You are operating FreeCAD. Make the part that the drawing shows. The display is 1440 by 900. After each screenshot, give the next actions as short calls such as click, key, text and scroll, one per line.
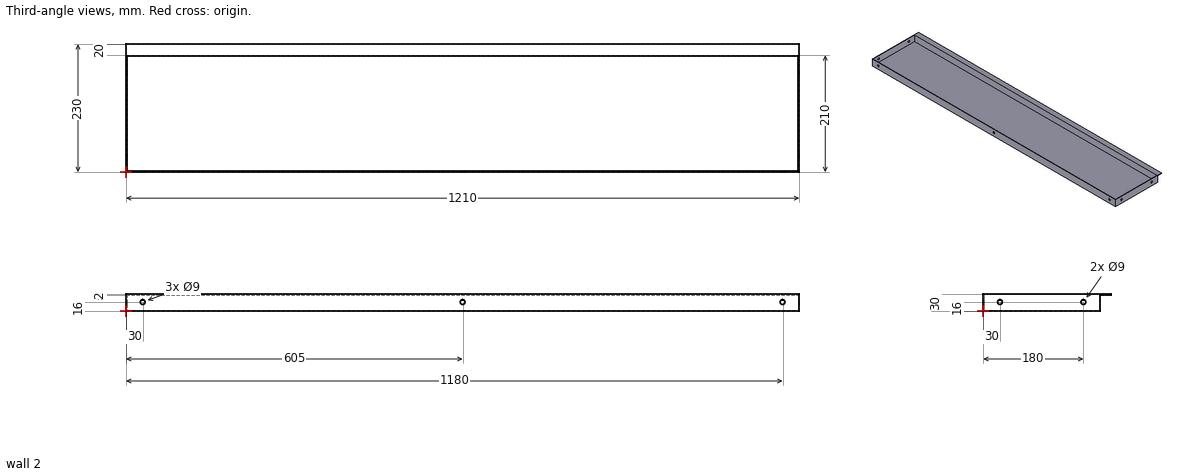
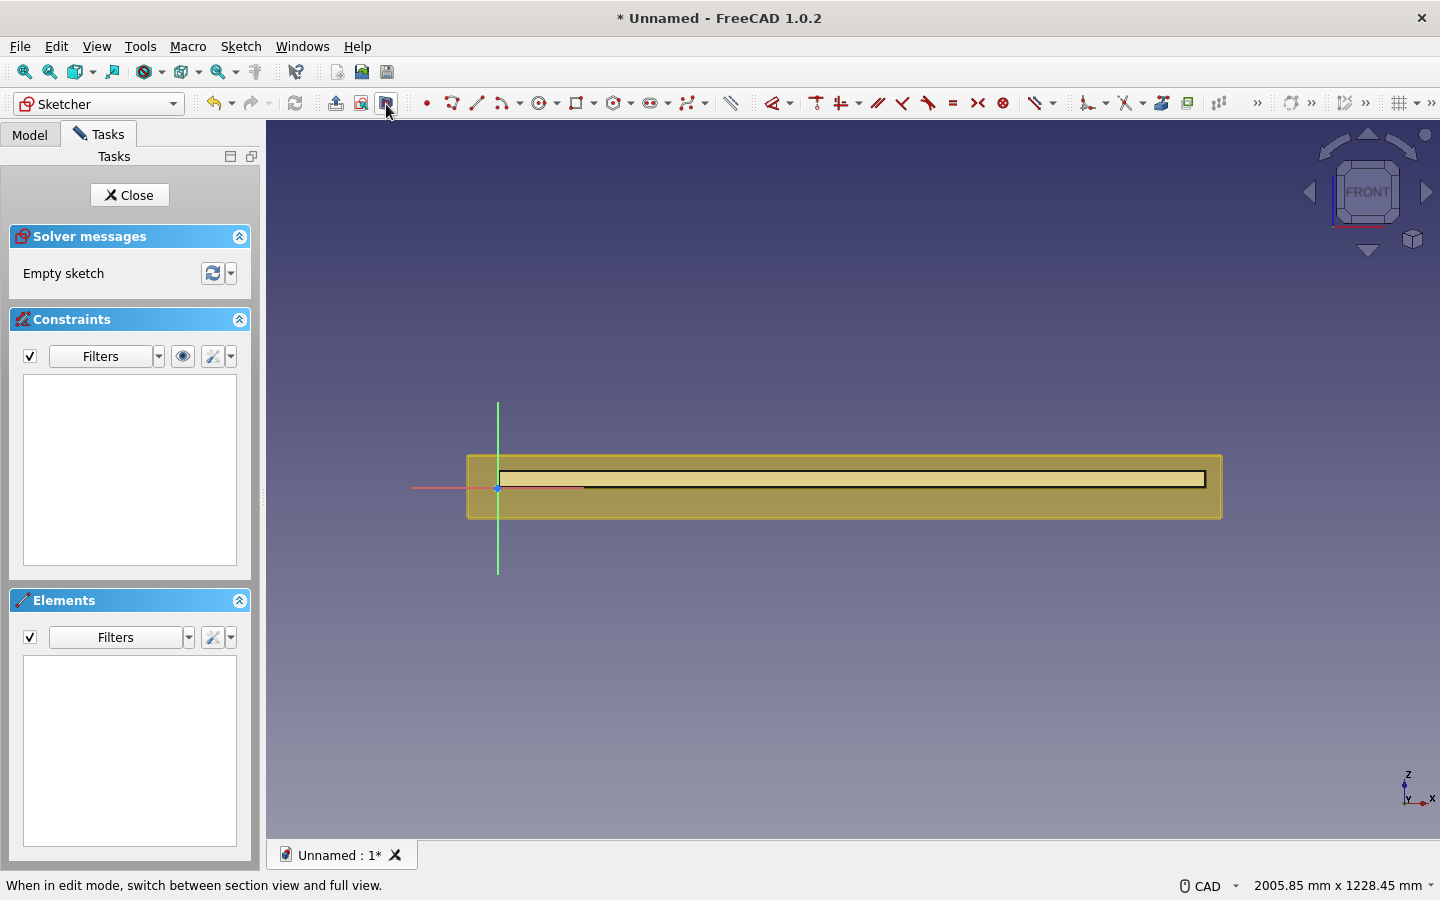
click(538, 104)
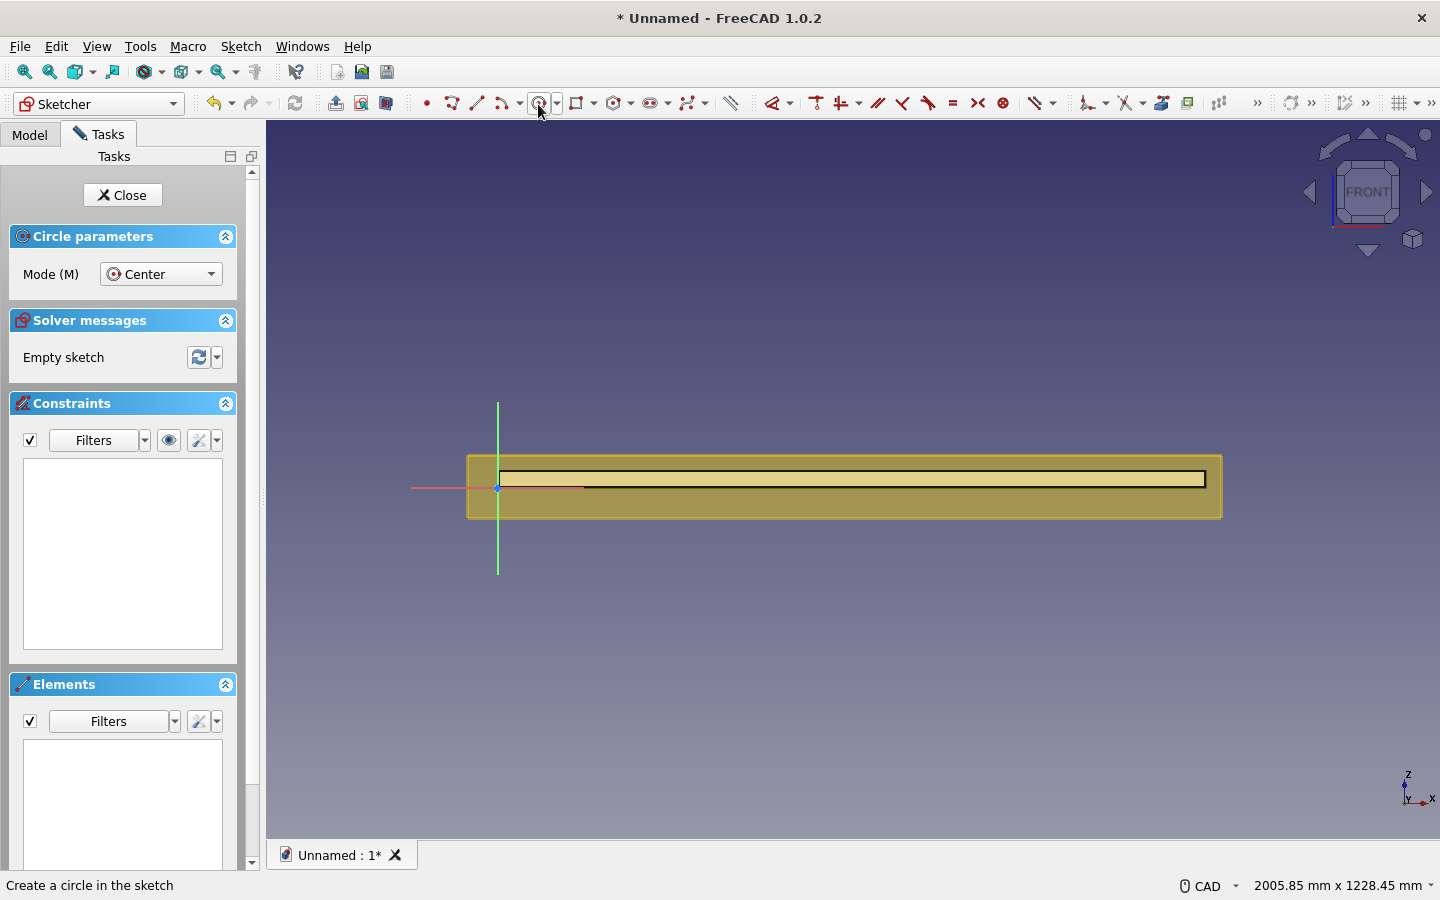
scroll(515, 479, up, 11)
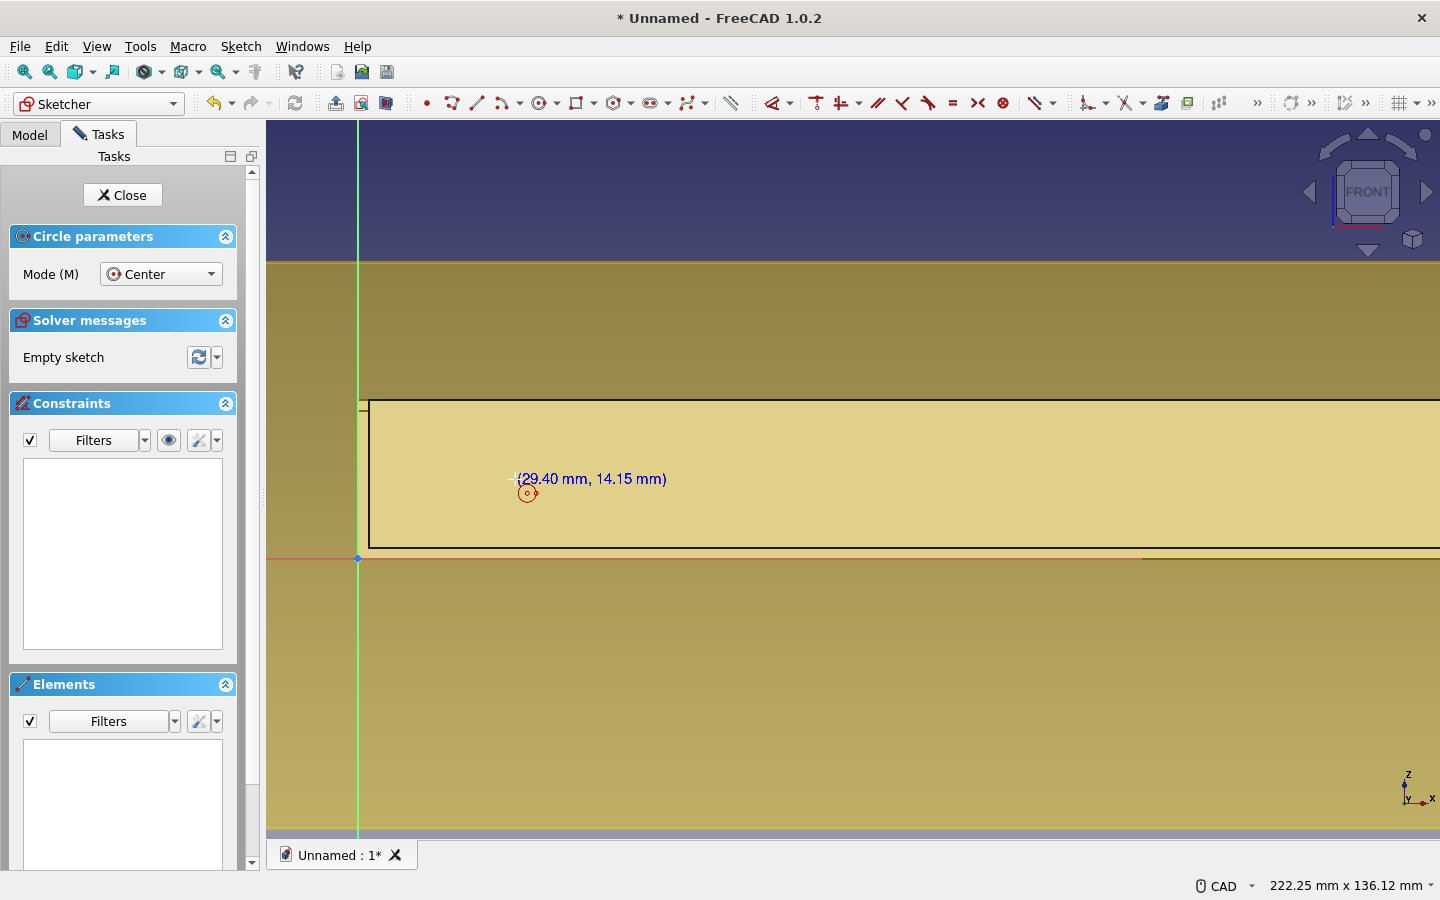
scroll(448, 476, down, 11)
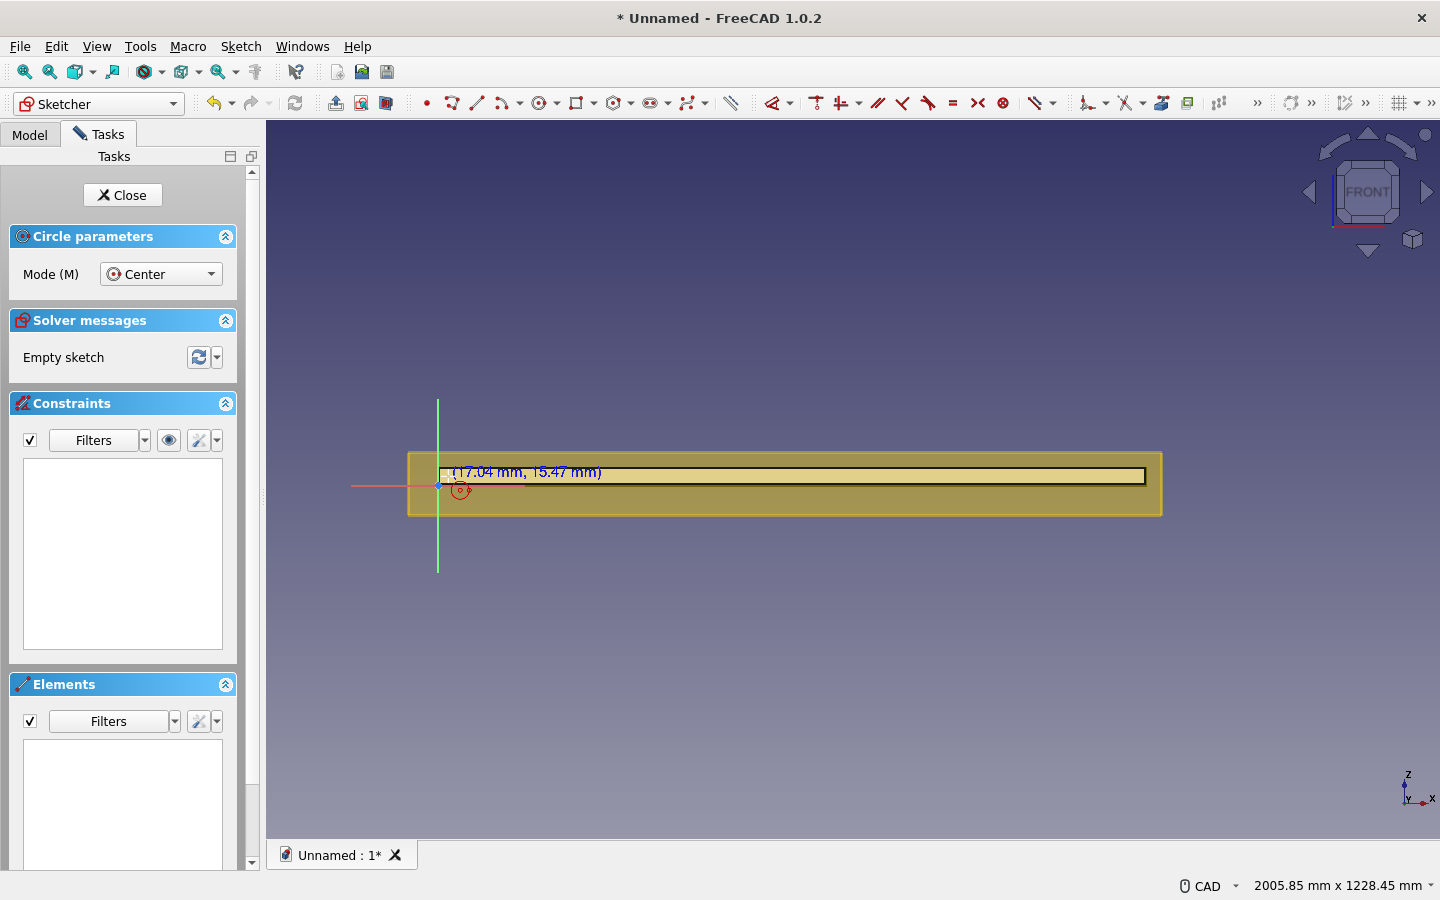
scroll(456, 476, up, 3)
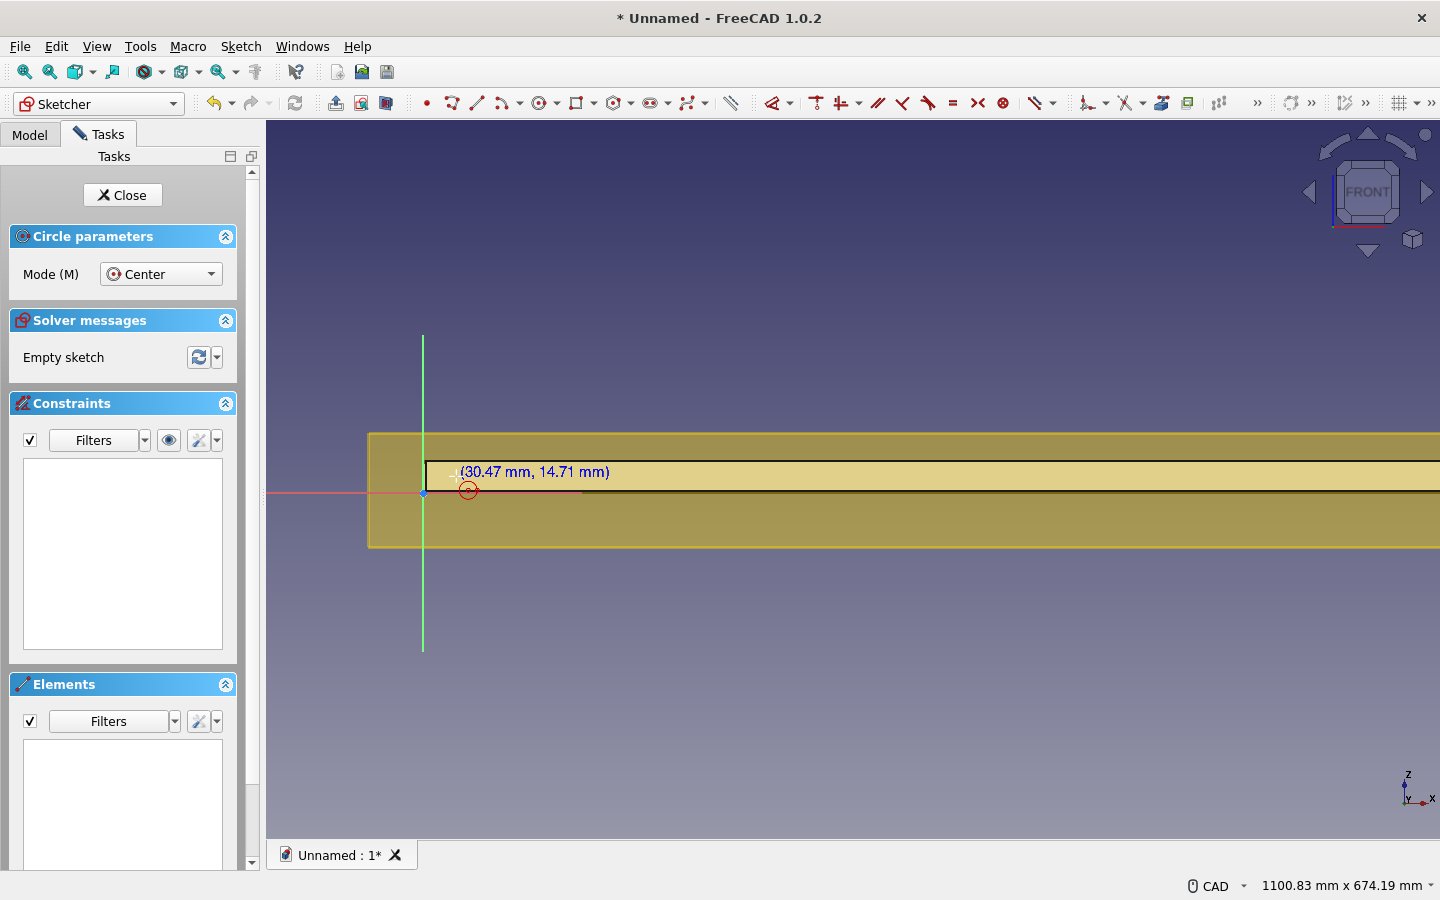
click(455, 476)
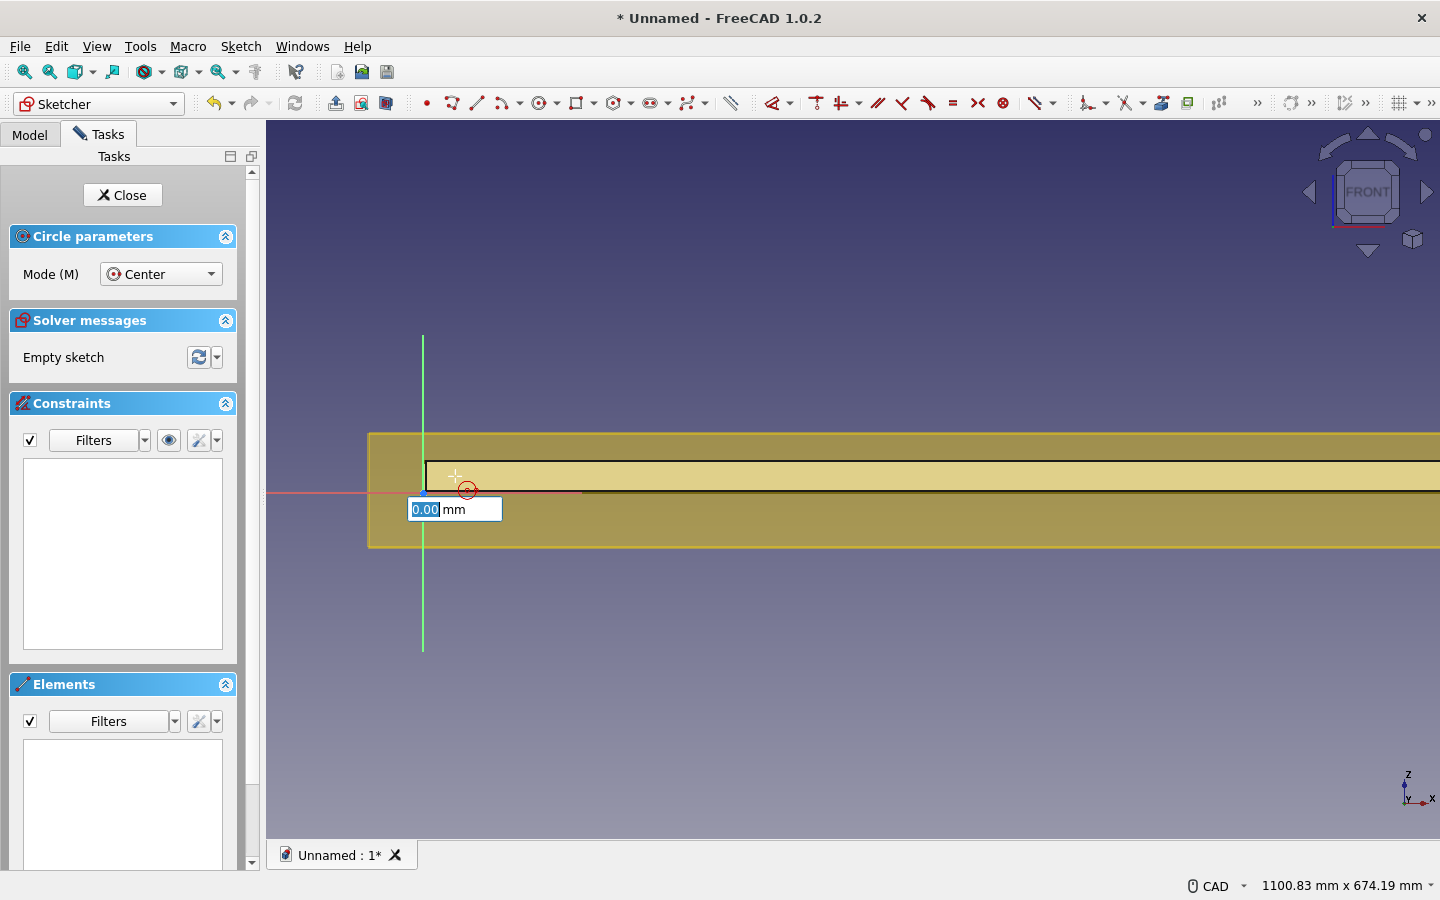
scroll(459, 473, up, 6)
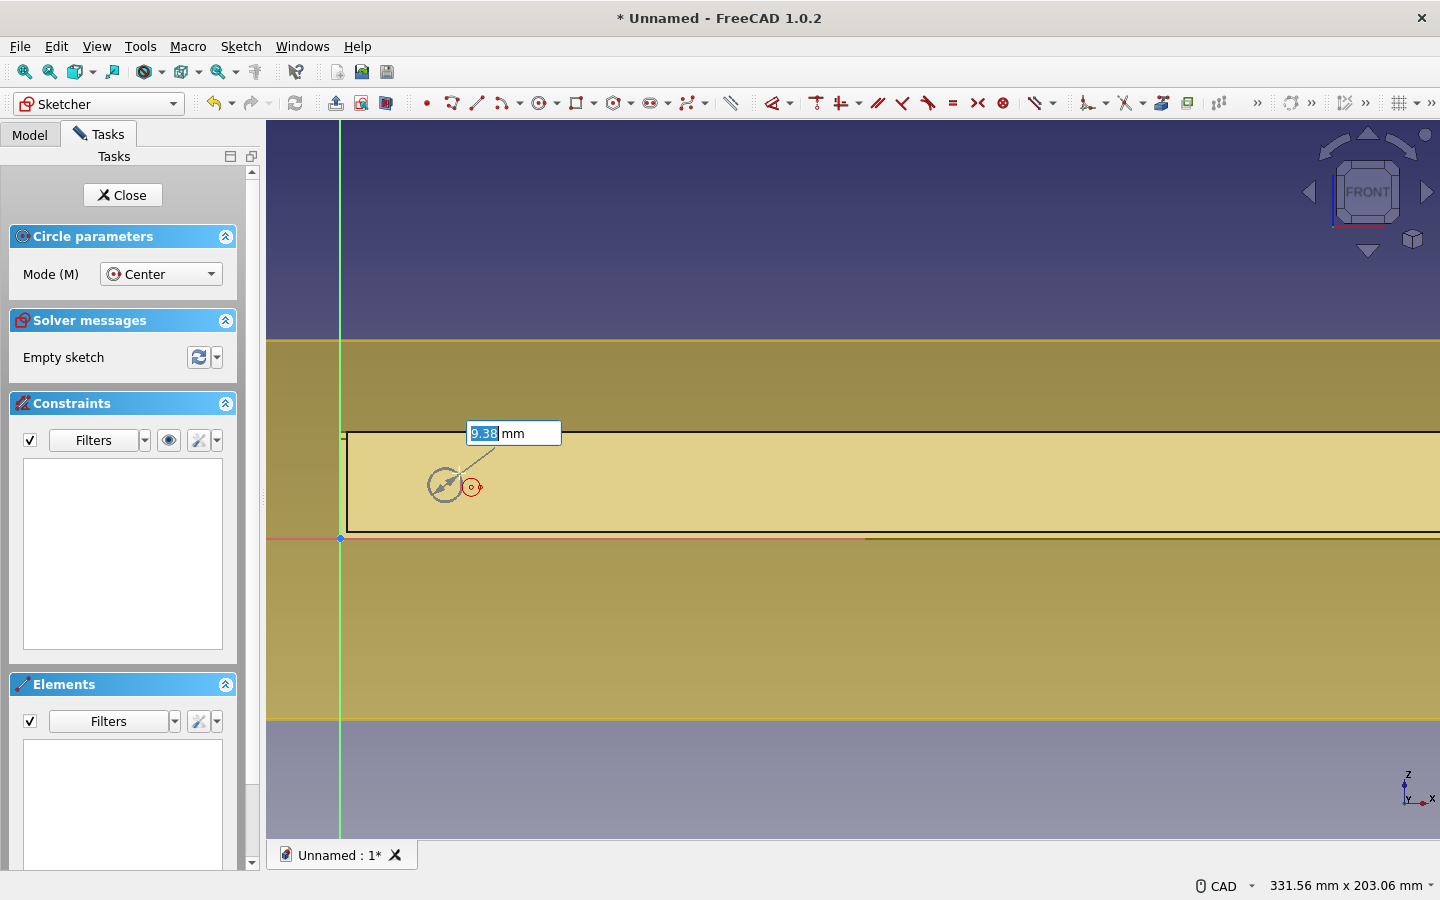
click(458, 471)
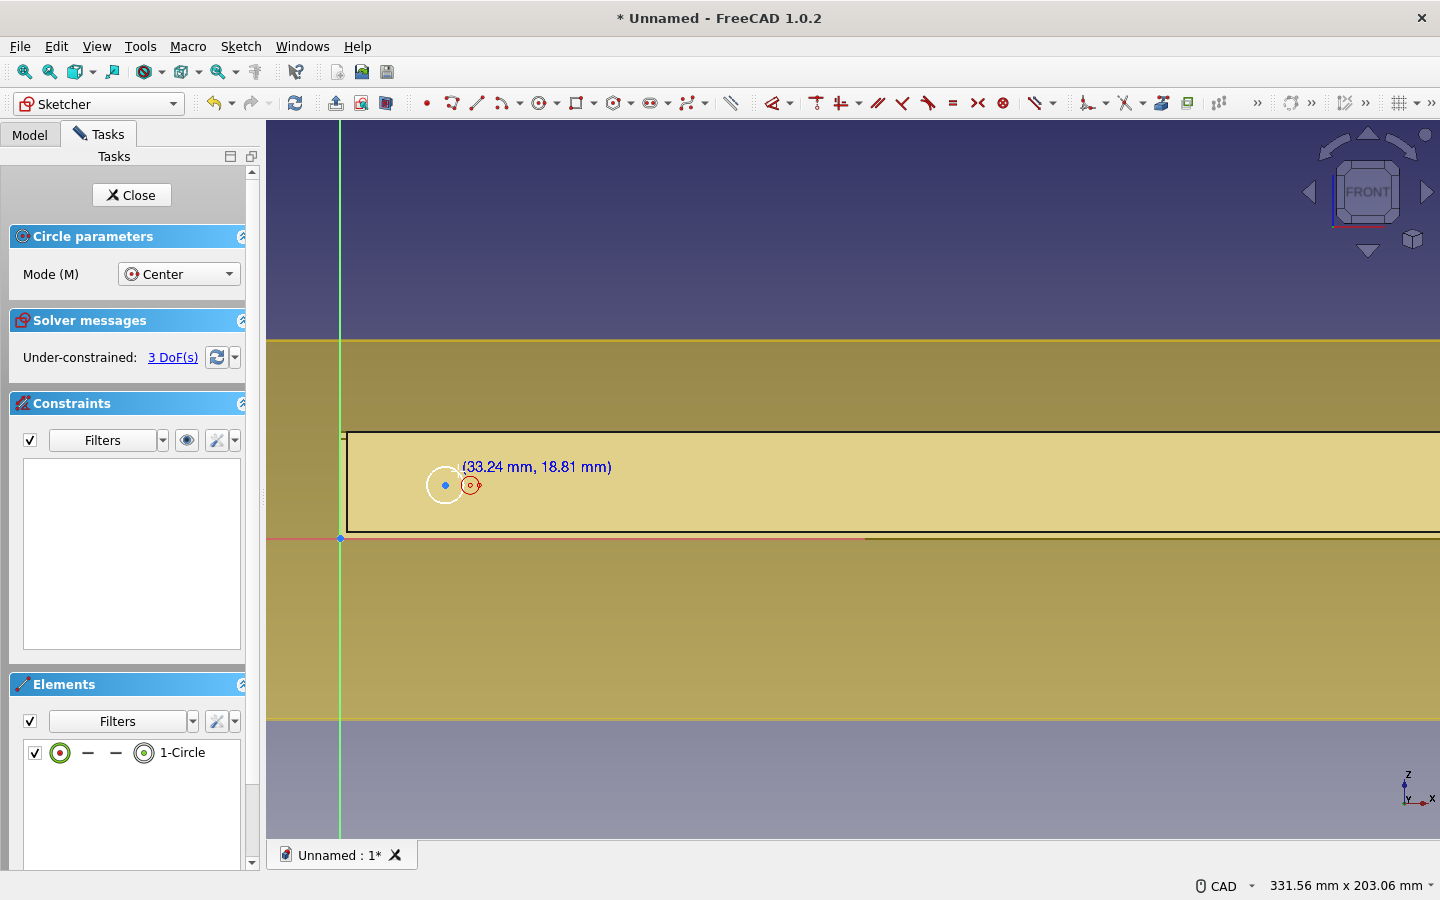
scroll(457, 475, down, 9)